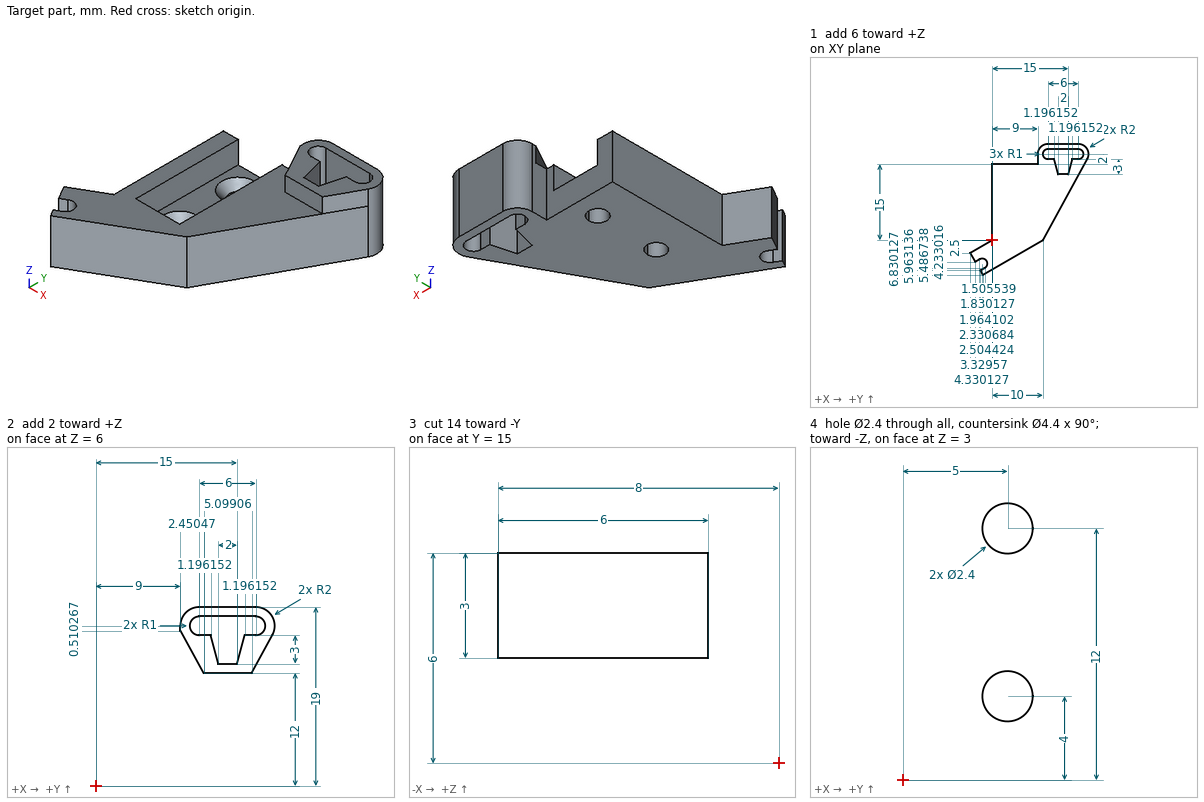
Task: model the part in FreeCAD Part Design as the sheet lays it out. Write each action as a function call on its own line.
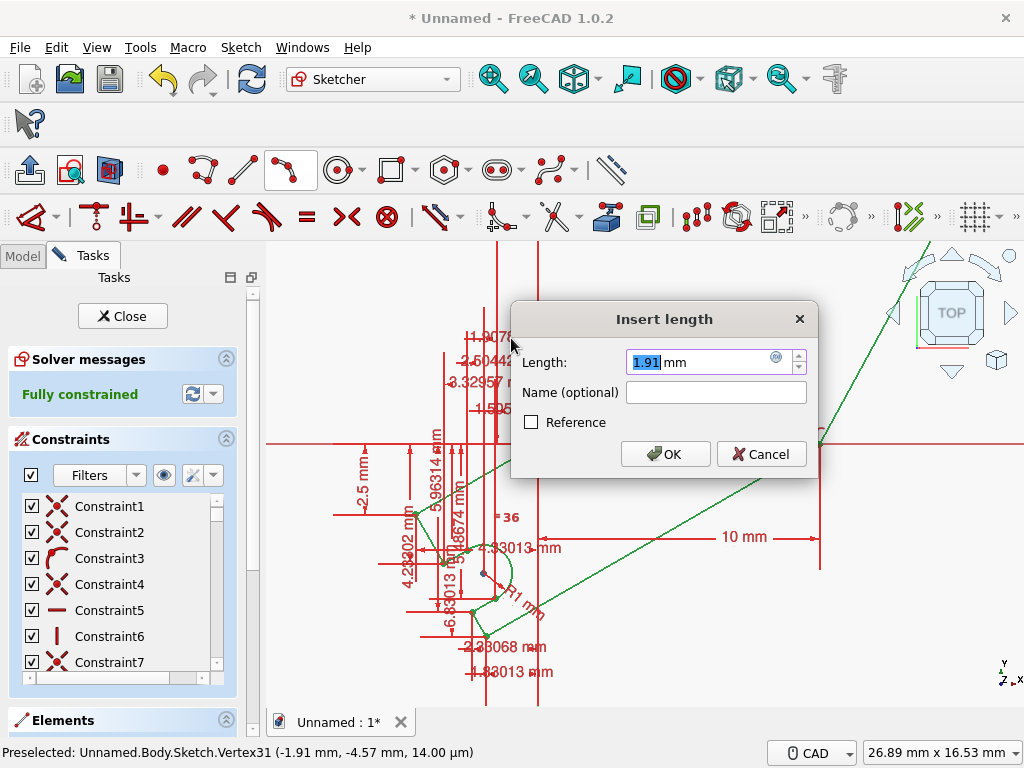
text(1.964102)
key(Return)
key(Escape)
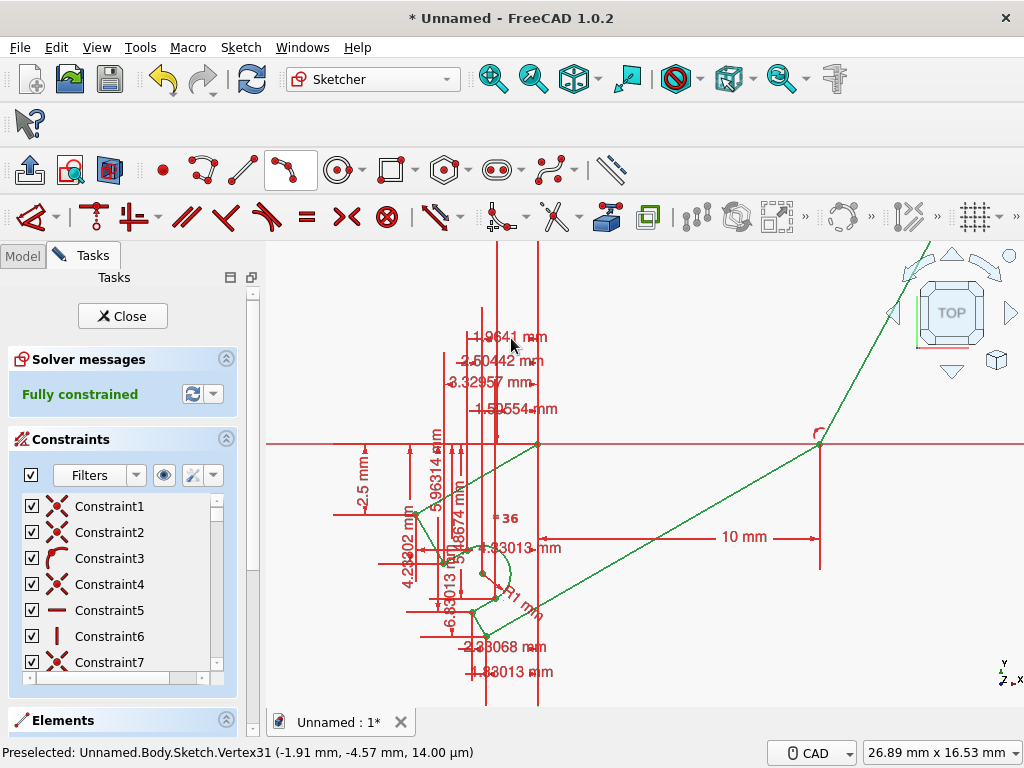
click(123, 316)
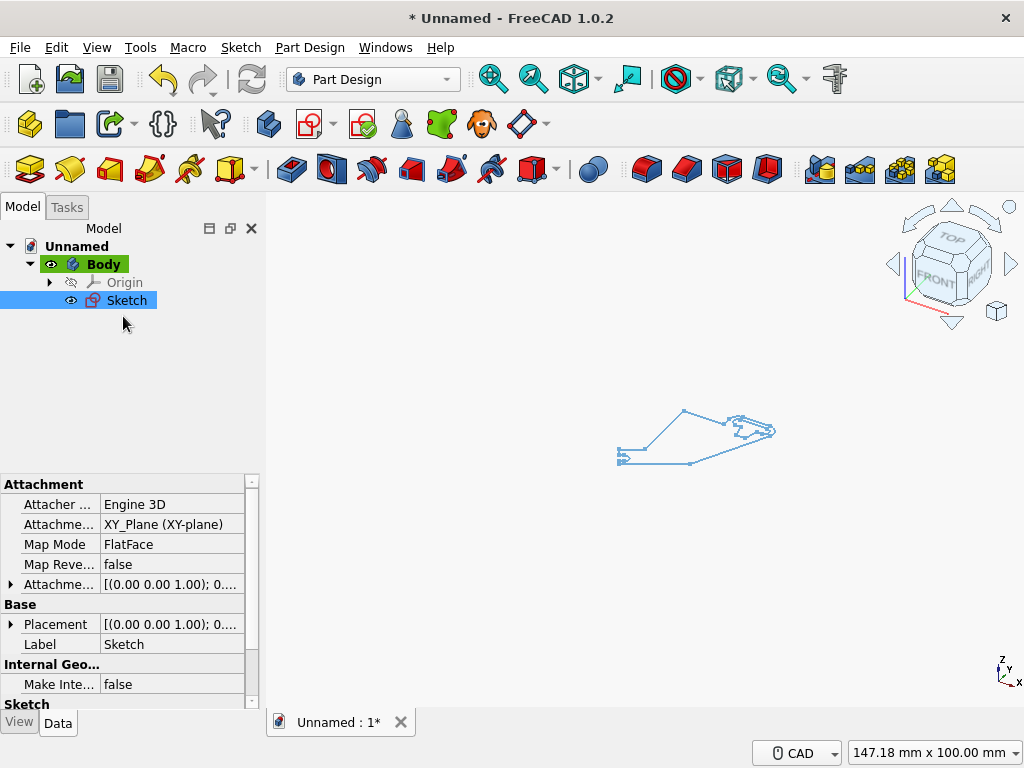
click(30, 170)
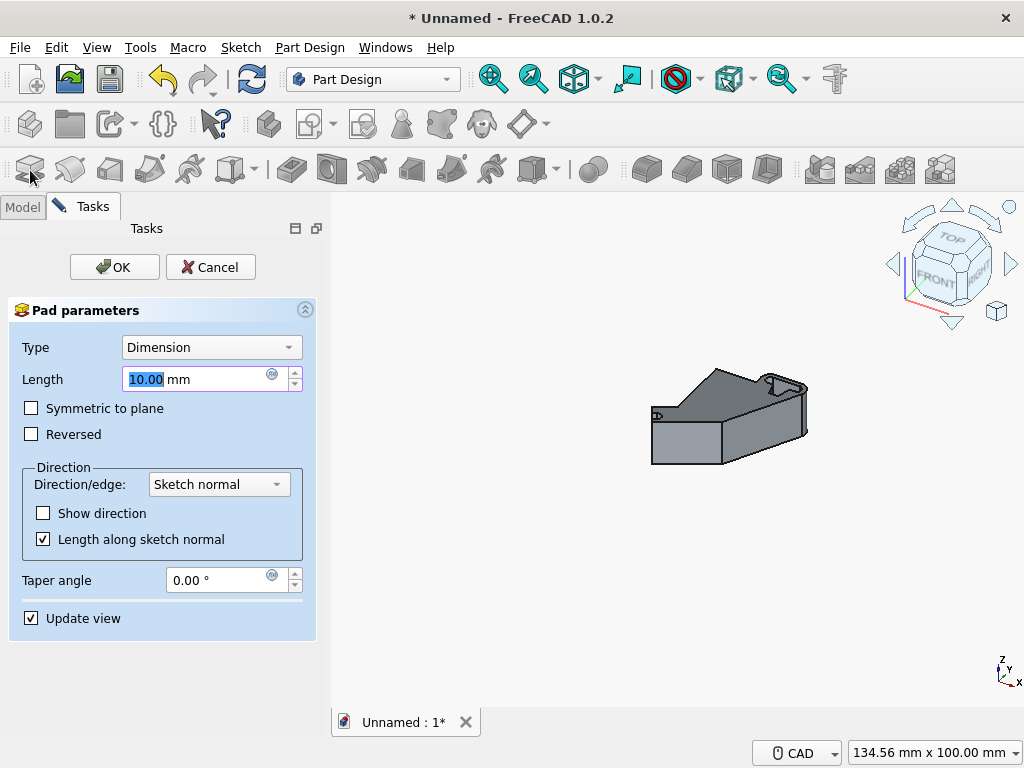
text(6)
key(Tab)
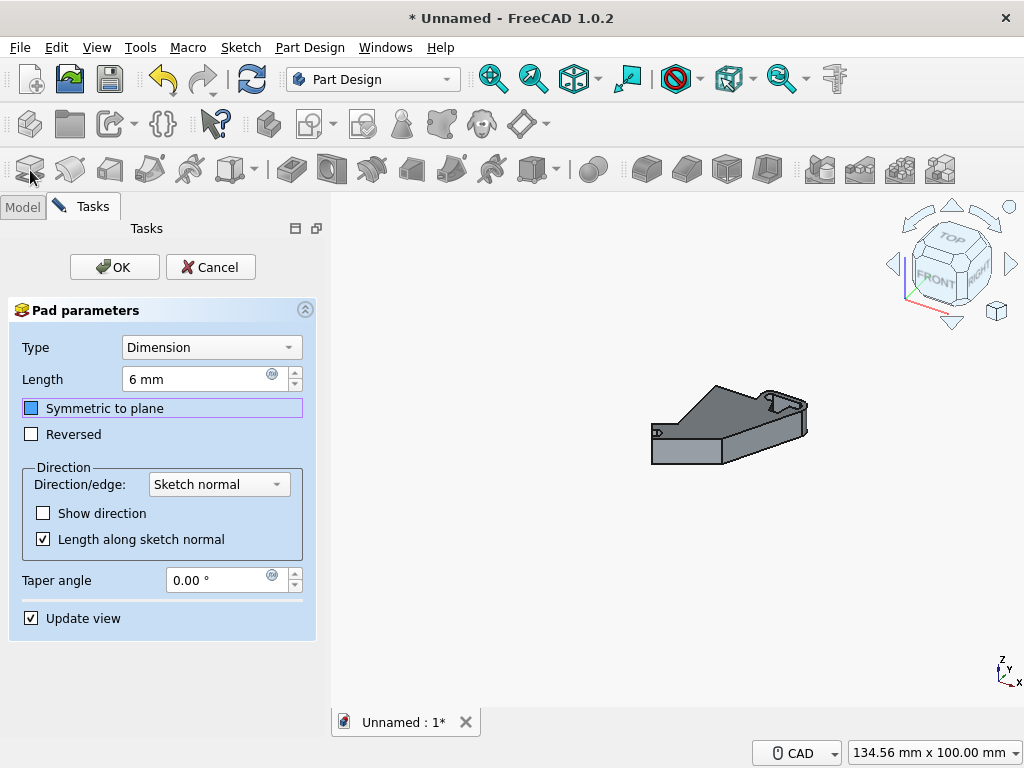
click(115, 267)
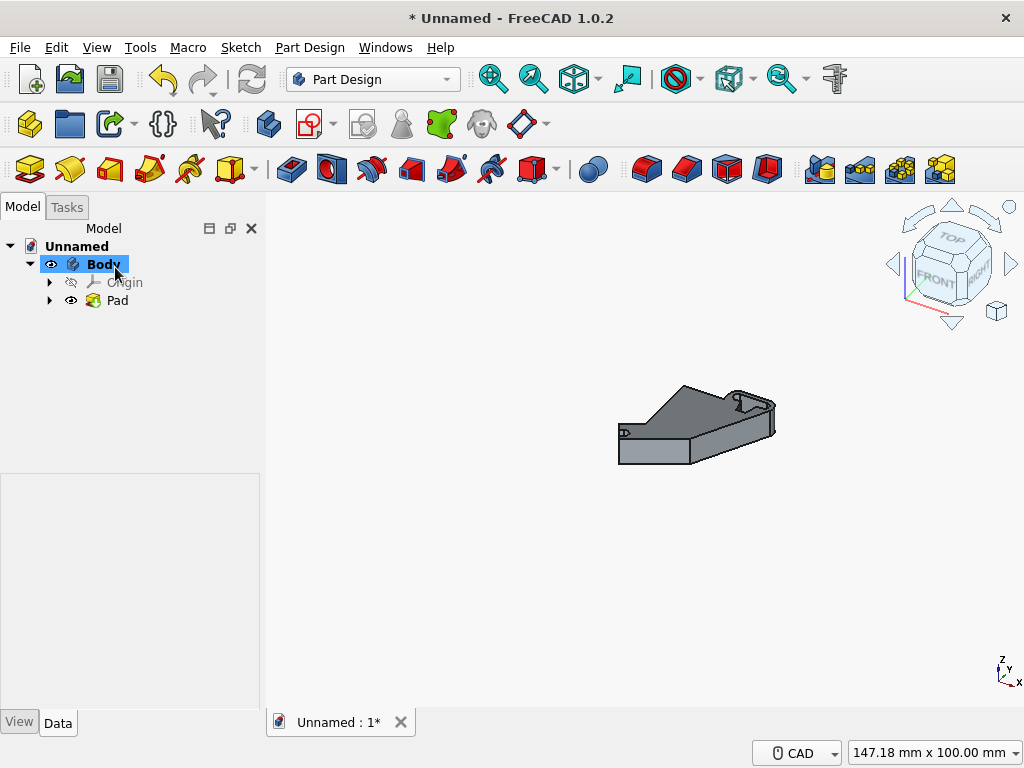
key(v)
key(f)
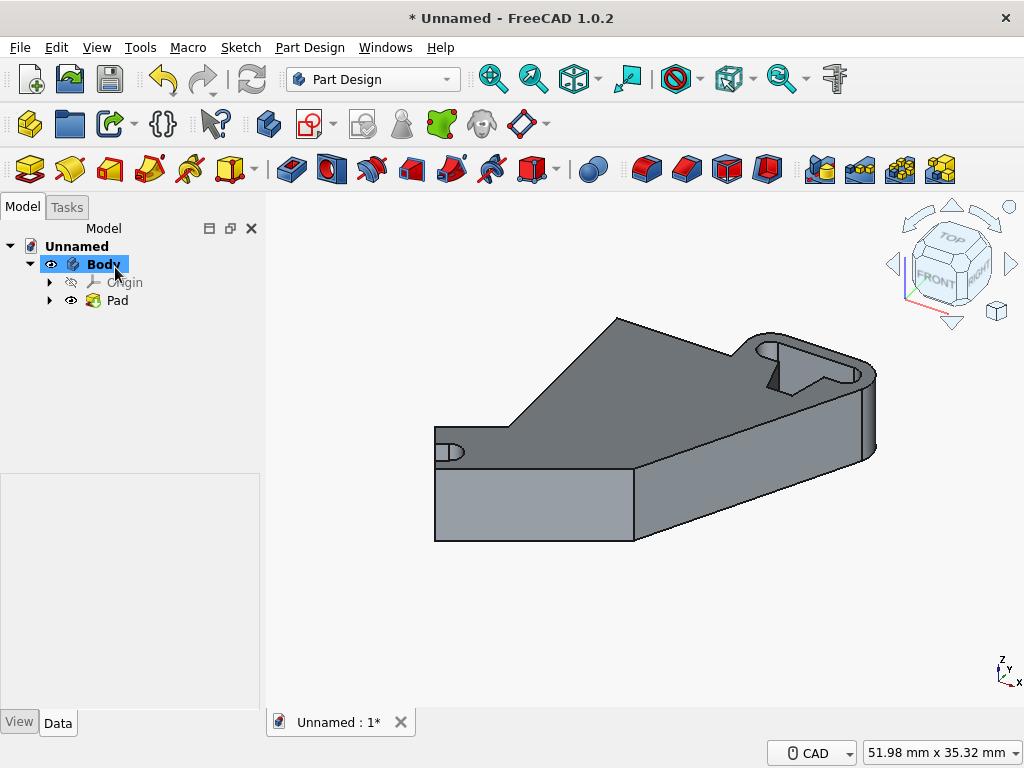
click(645, 413)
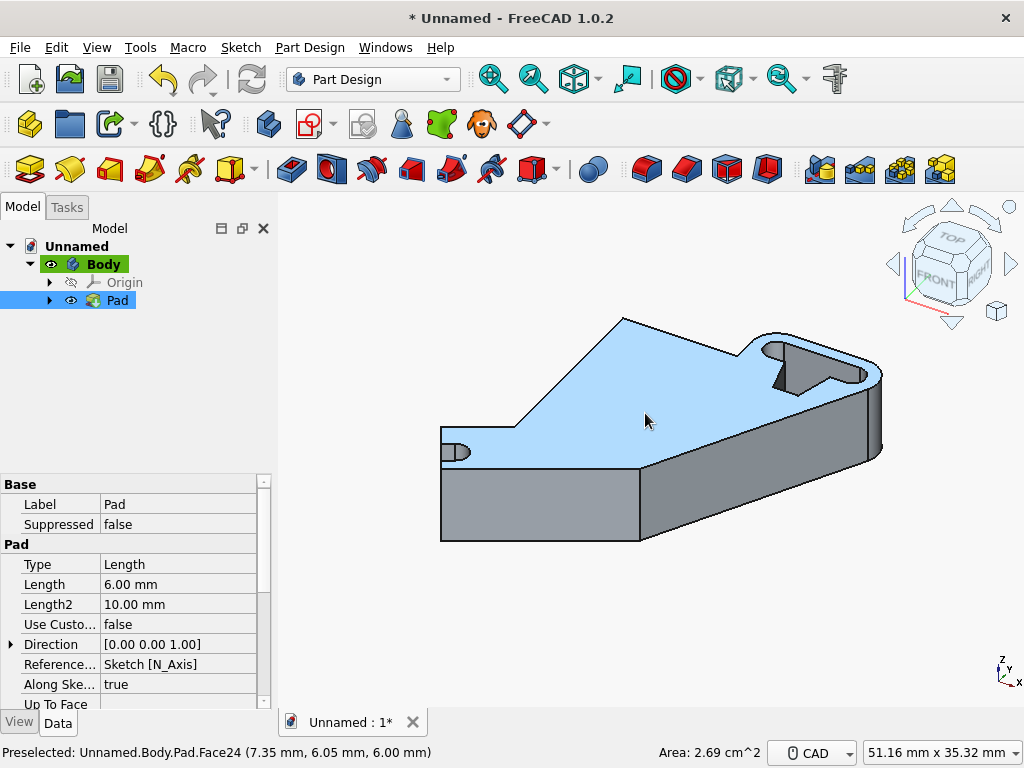
click(310, 124)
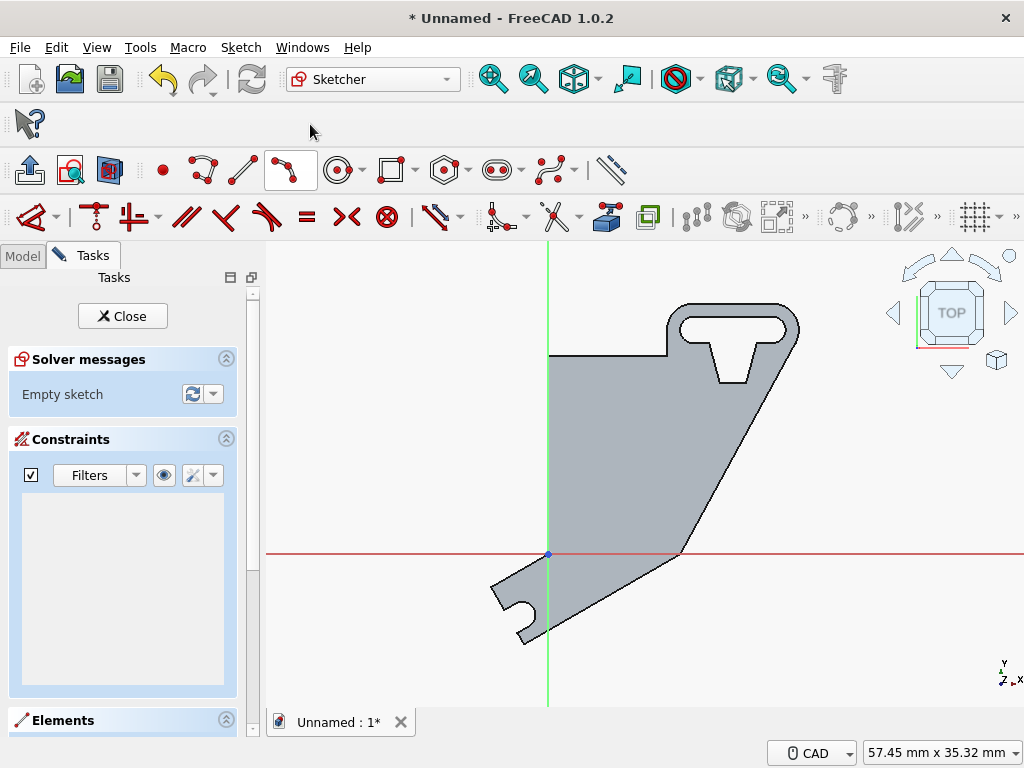
key(g)
key(l)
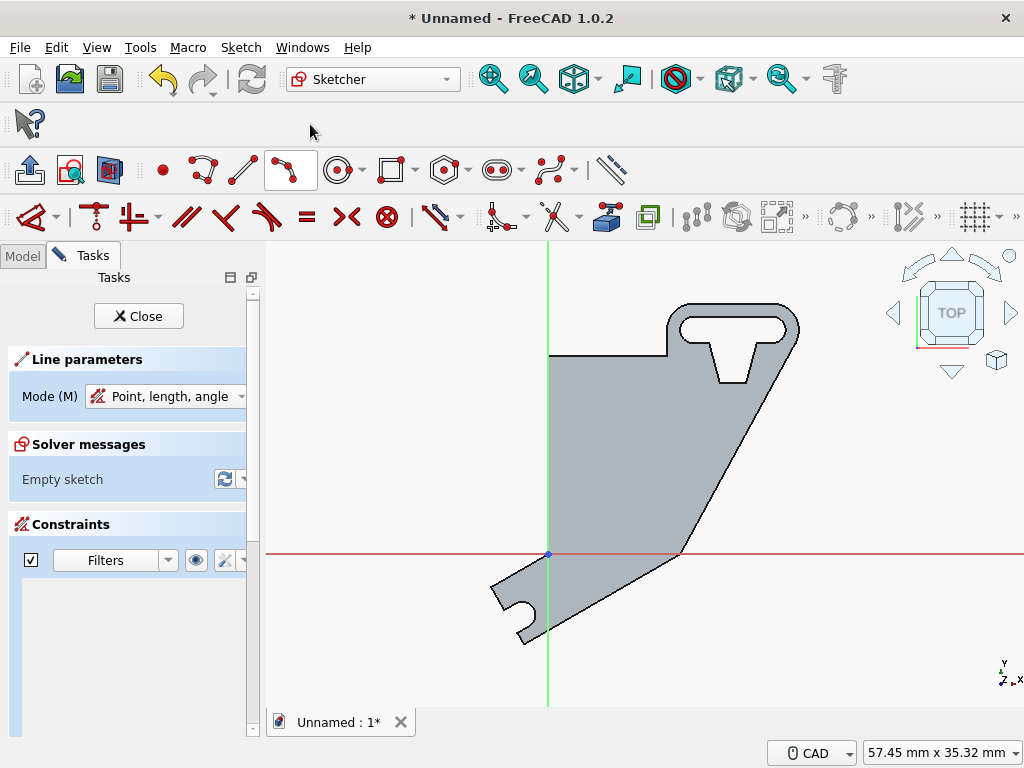
click(773, 304)
click(693, 304)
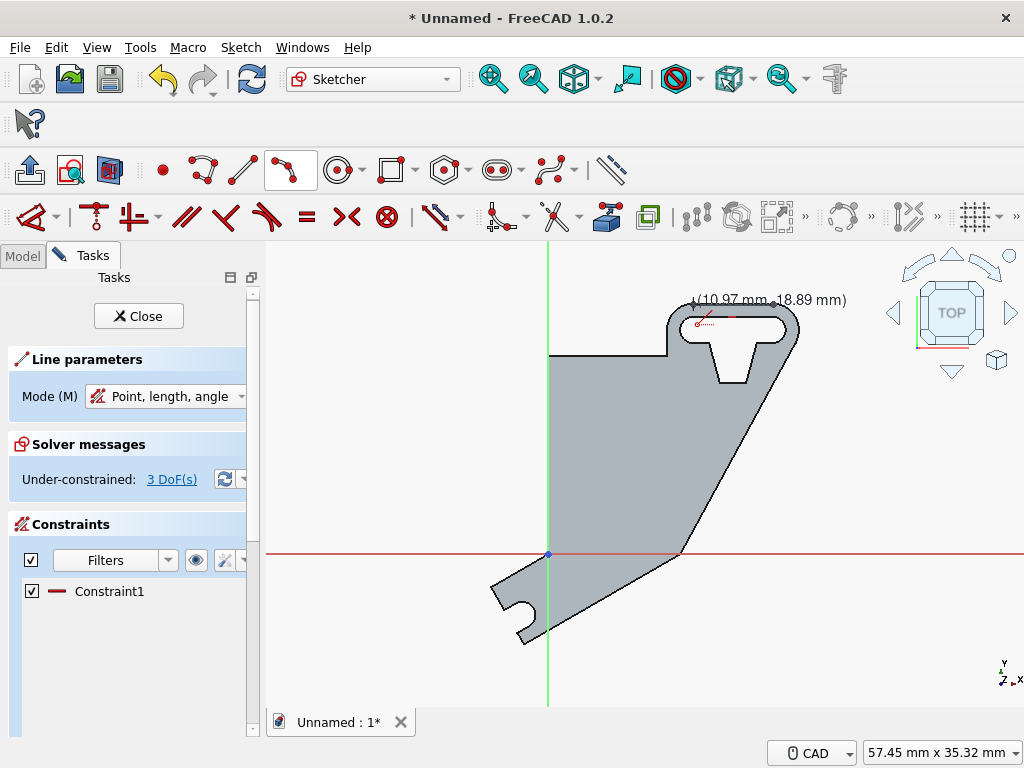
click(204, 170)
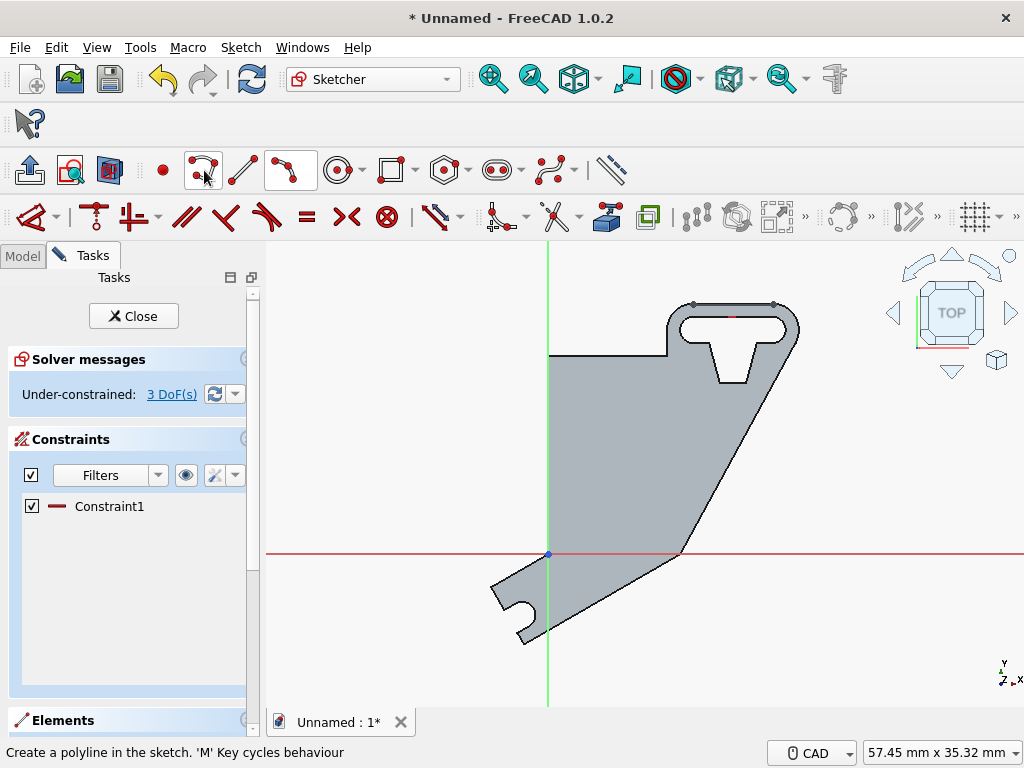
click(667, 330)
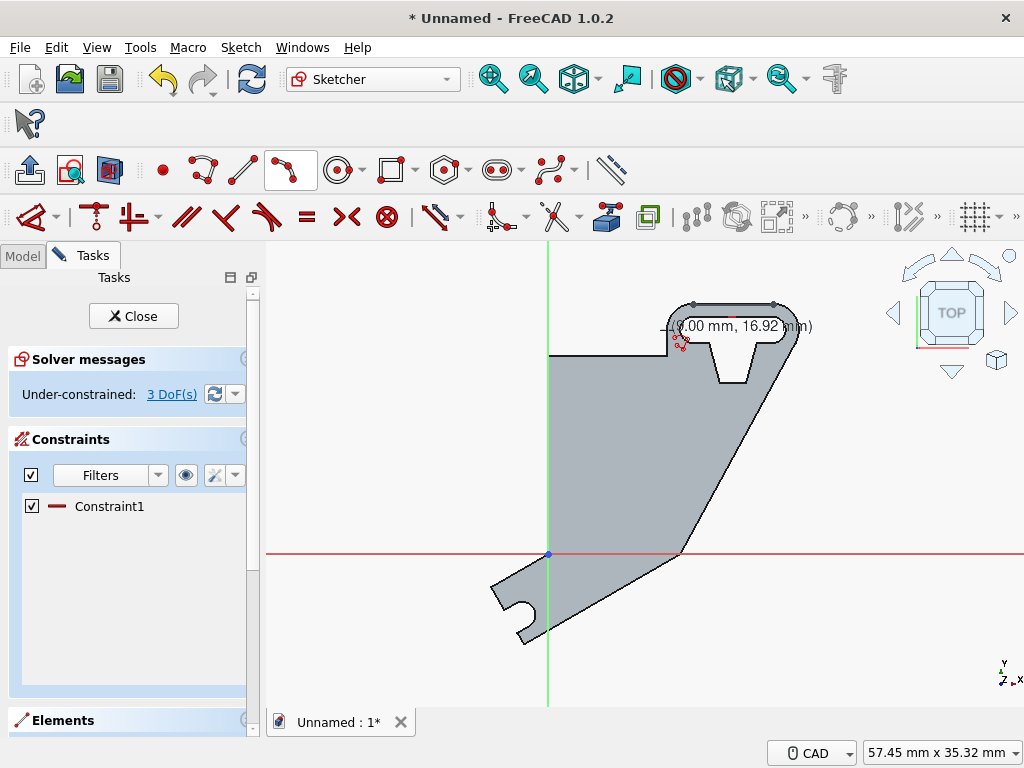
scroll(667, 337, up, 5)